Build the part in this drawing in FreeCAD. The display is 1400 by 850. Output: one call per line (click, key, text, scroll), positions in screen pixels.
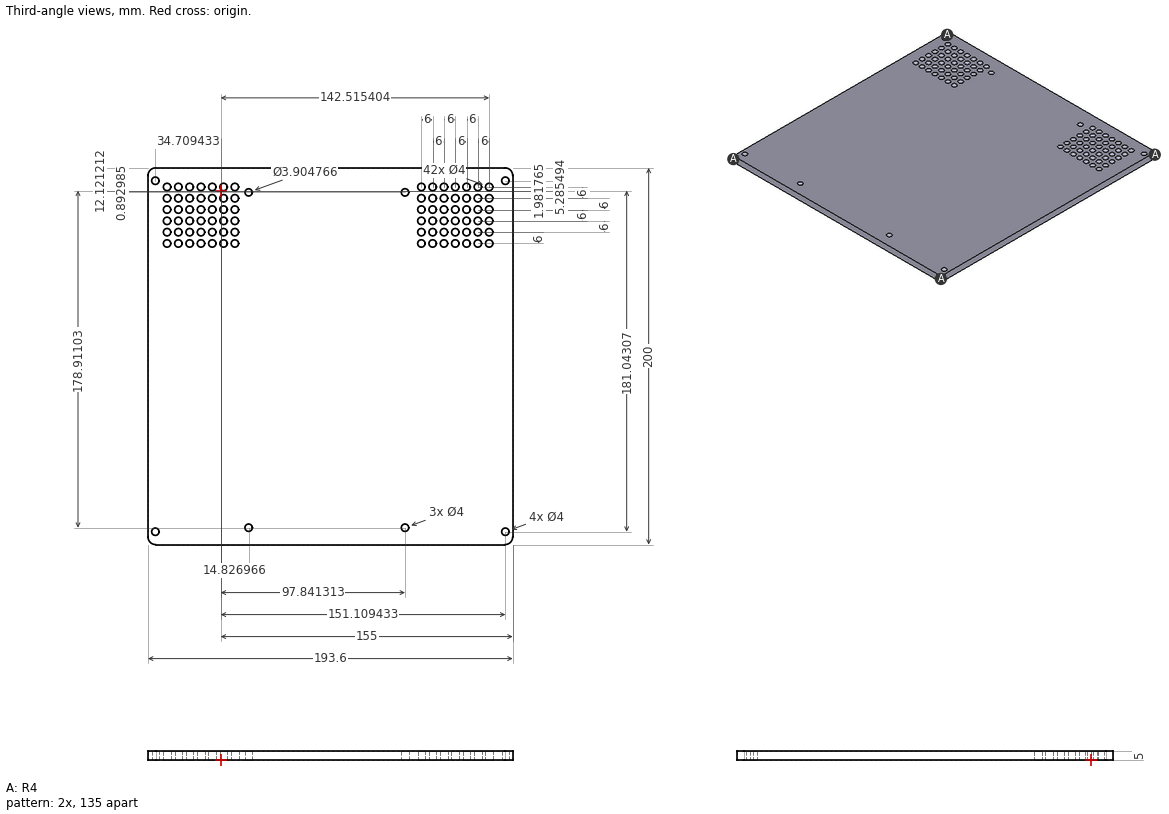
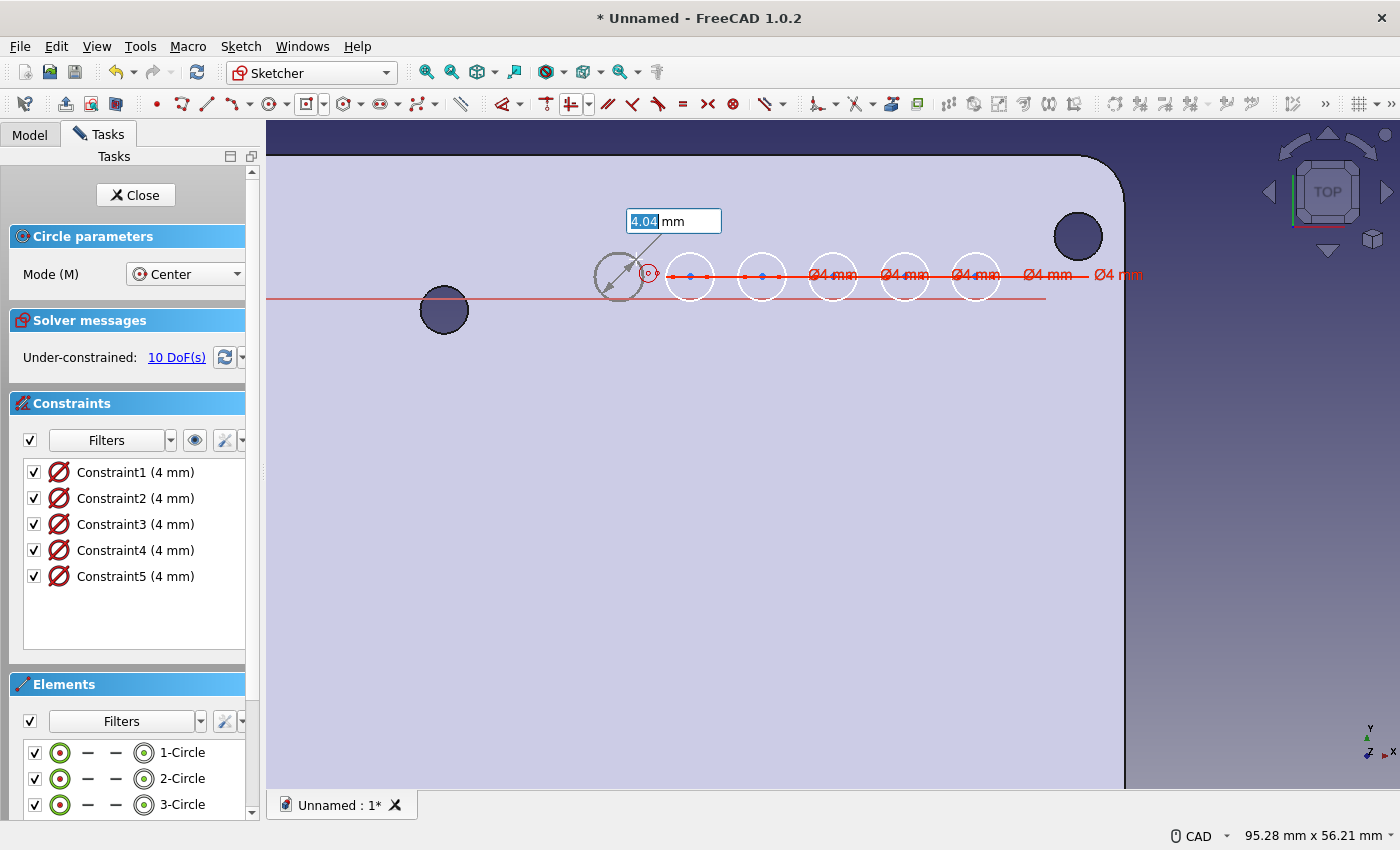
text(4)
key(Return)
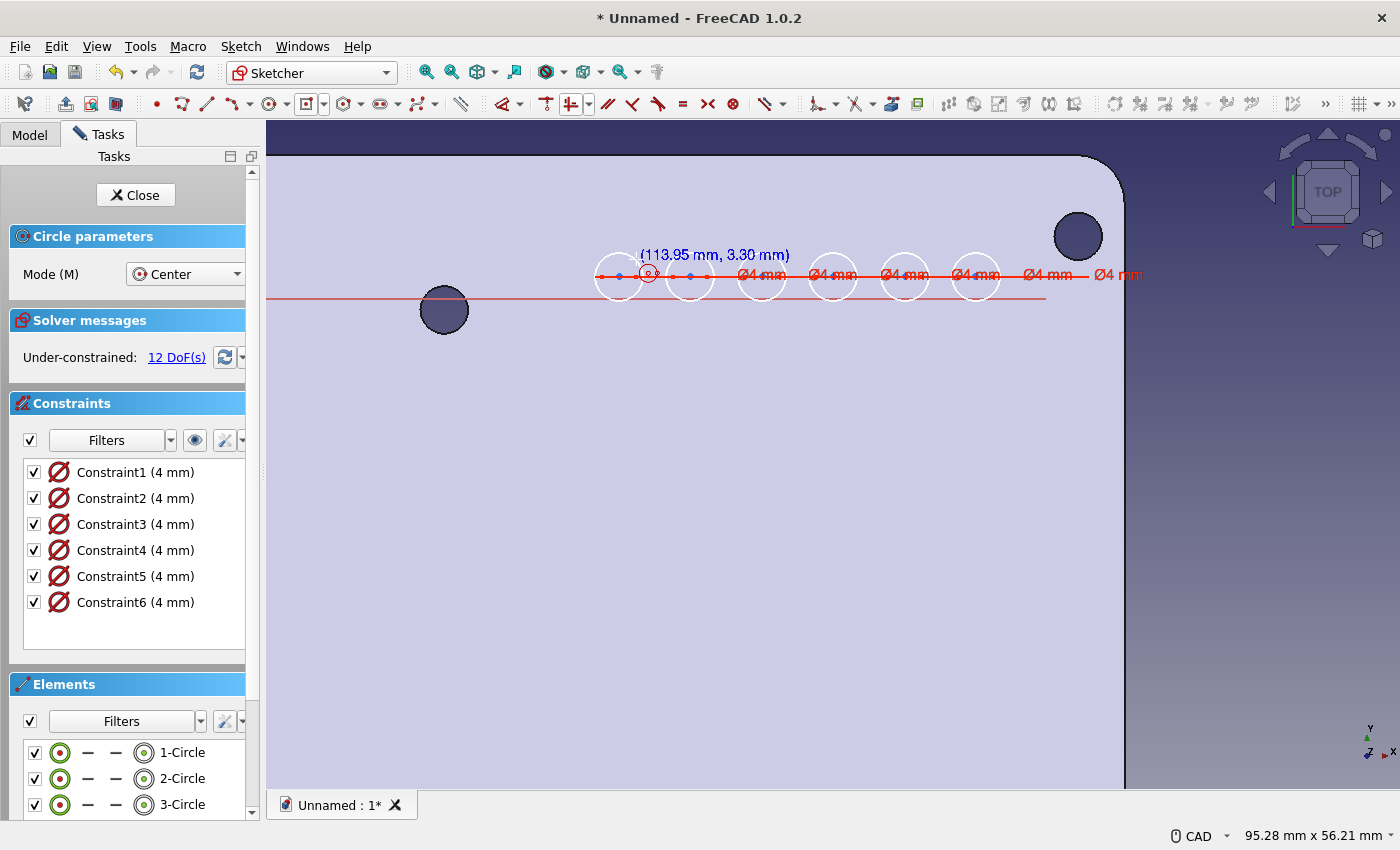
click(548, 276)
move(564, 259)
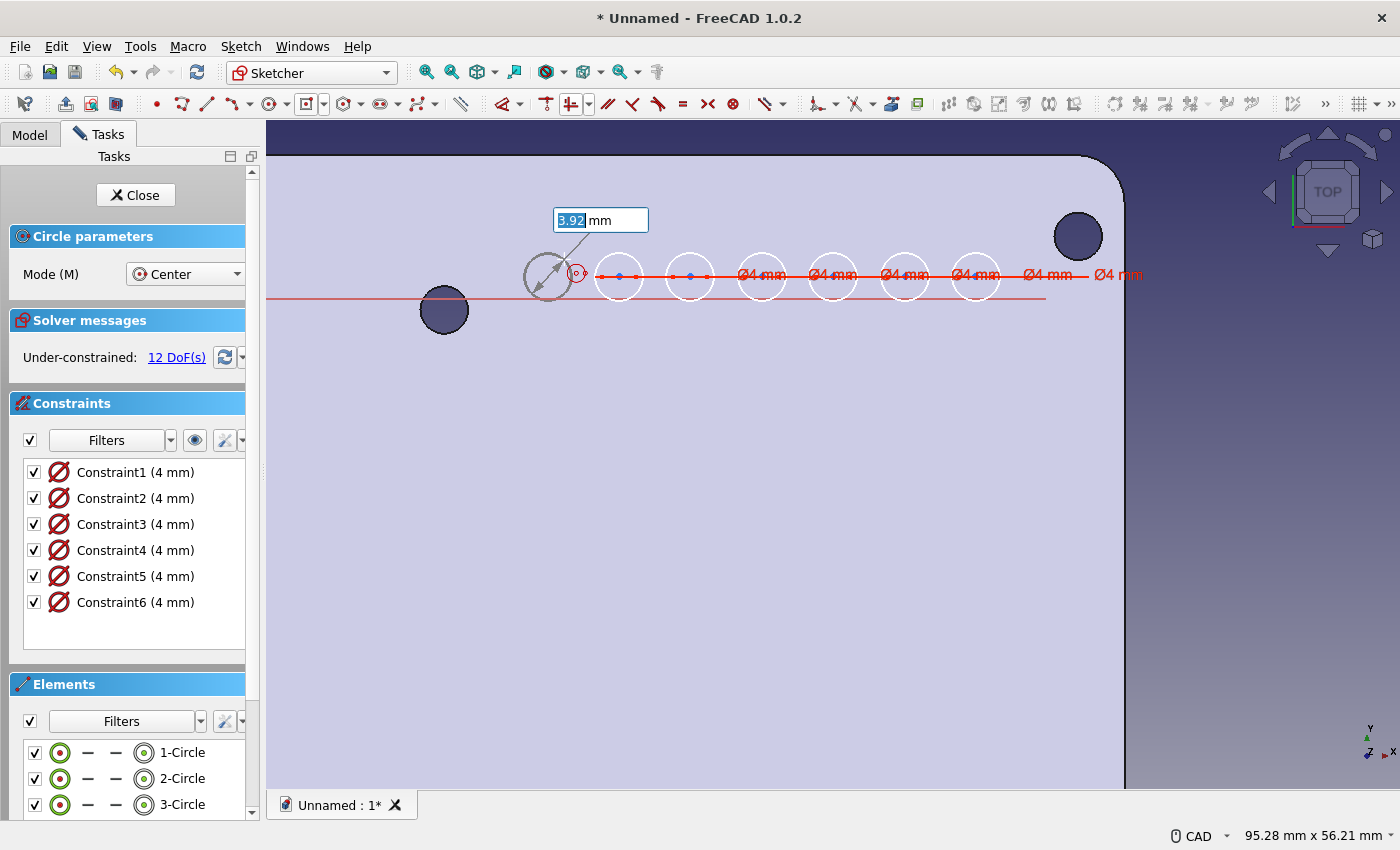
text(4)
key(Return)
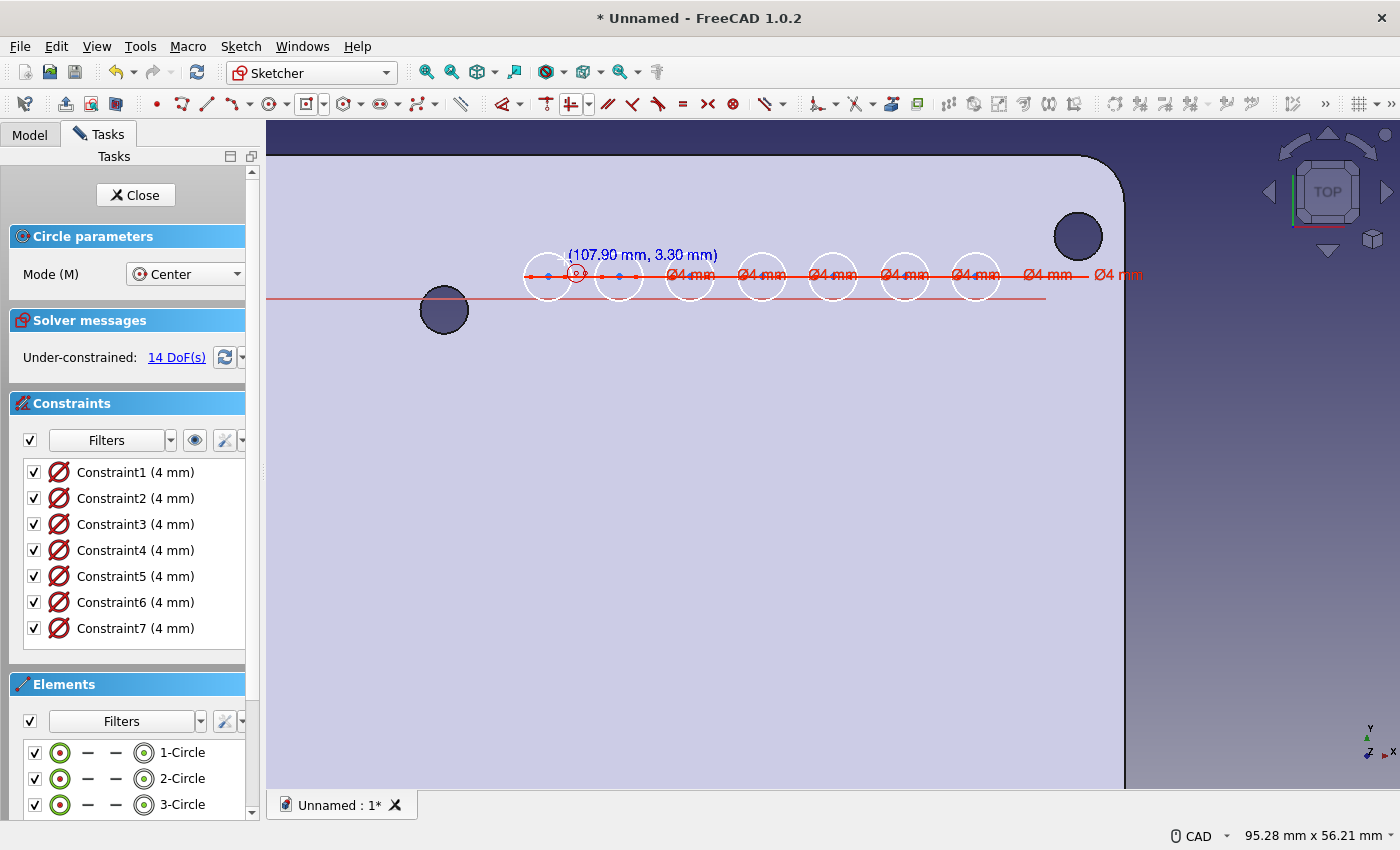
click(905, 347)
move(921, 330)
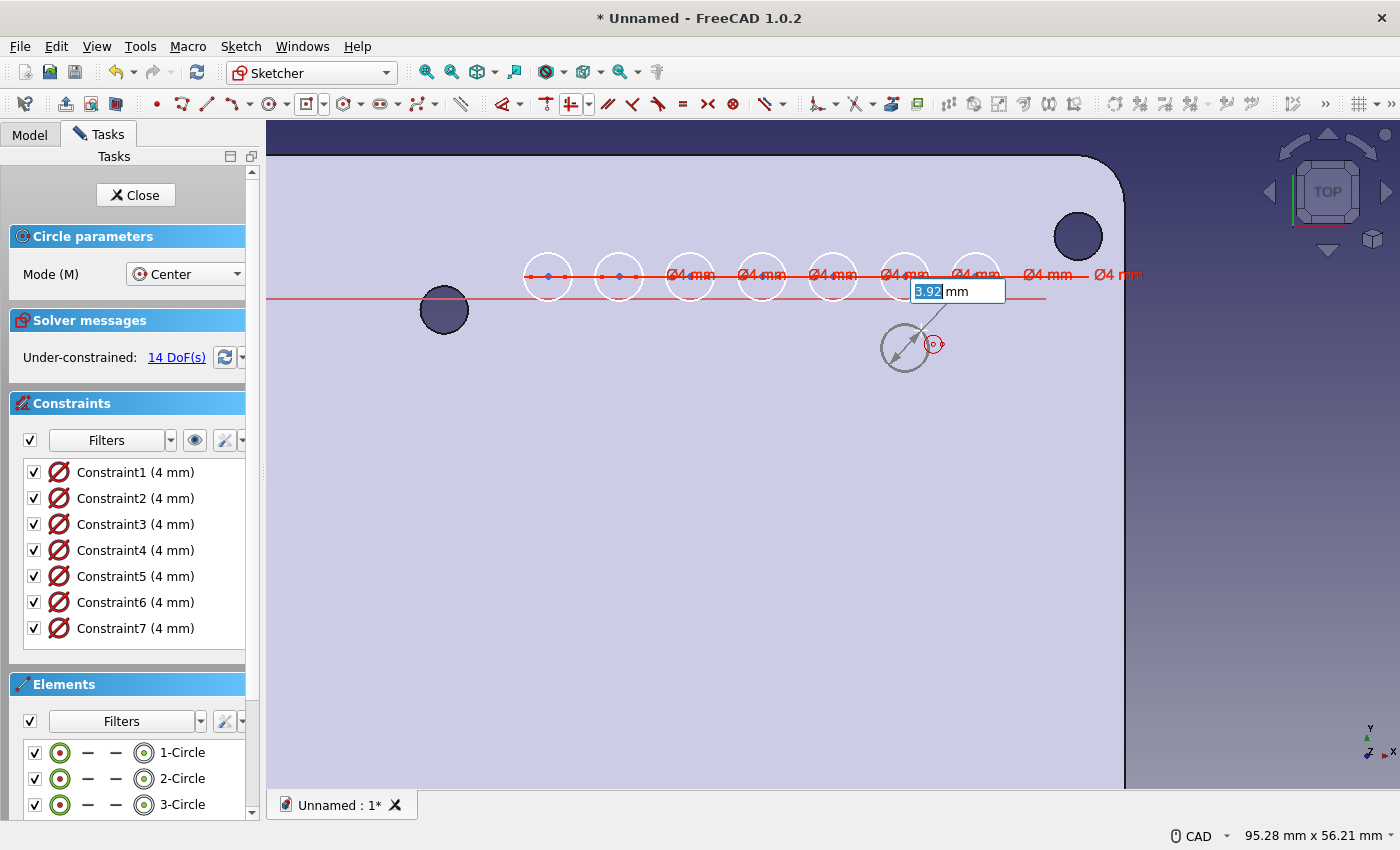
text(4)
key(Return)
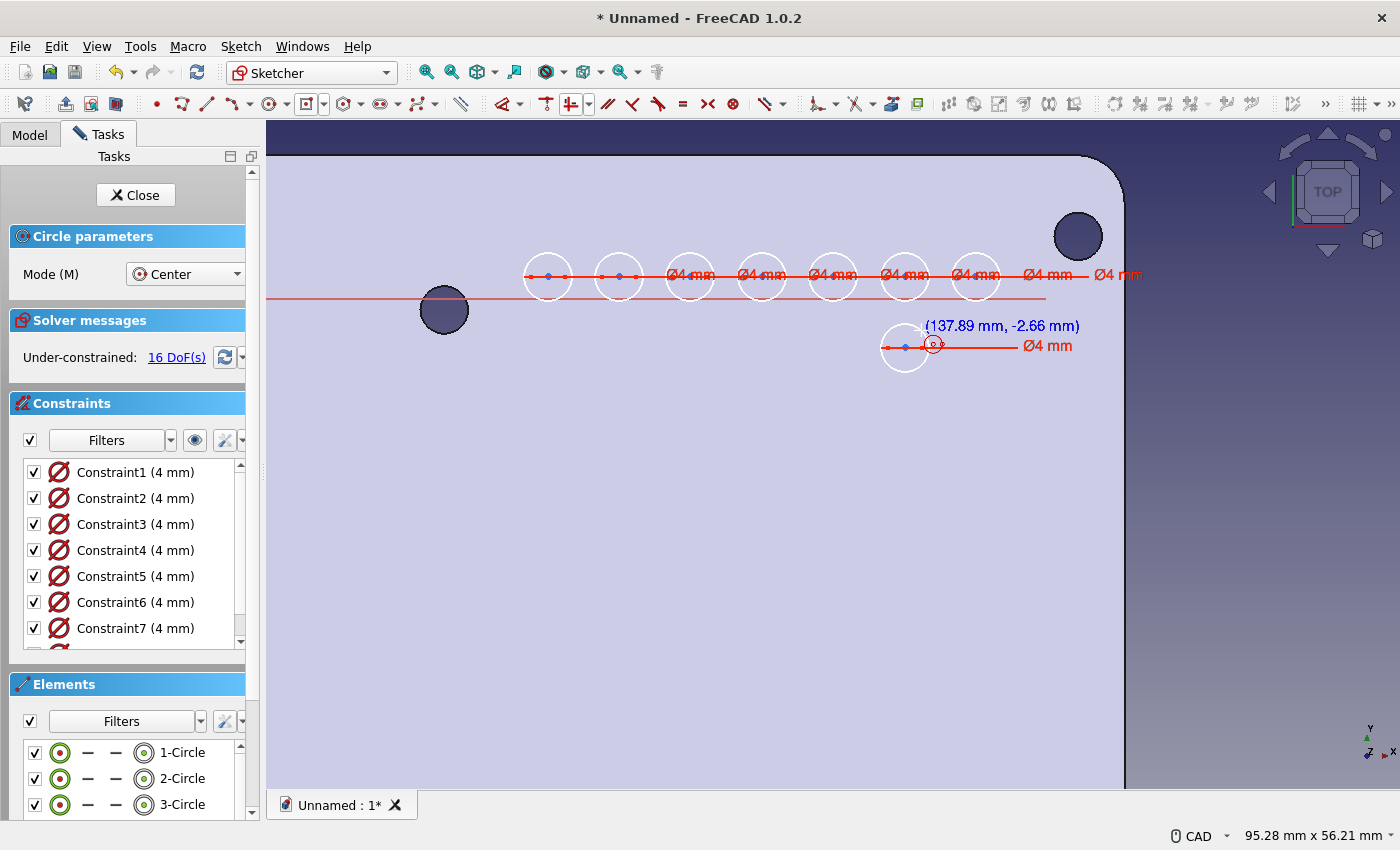
click(833, 347)
move(850, 330)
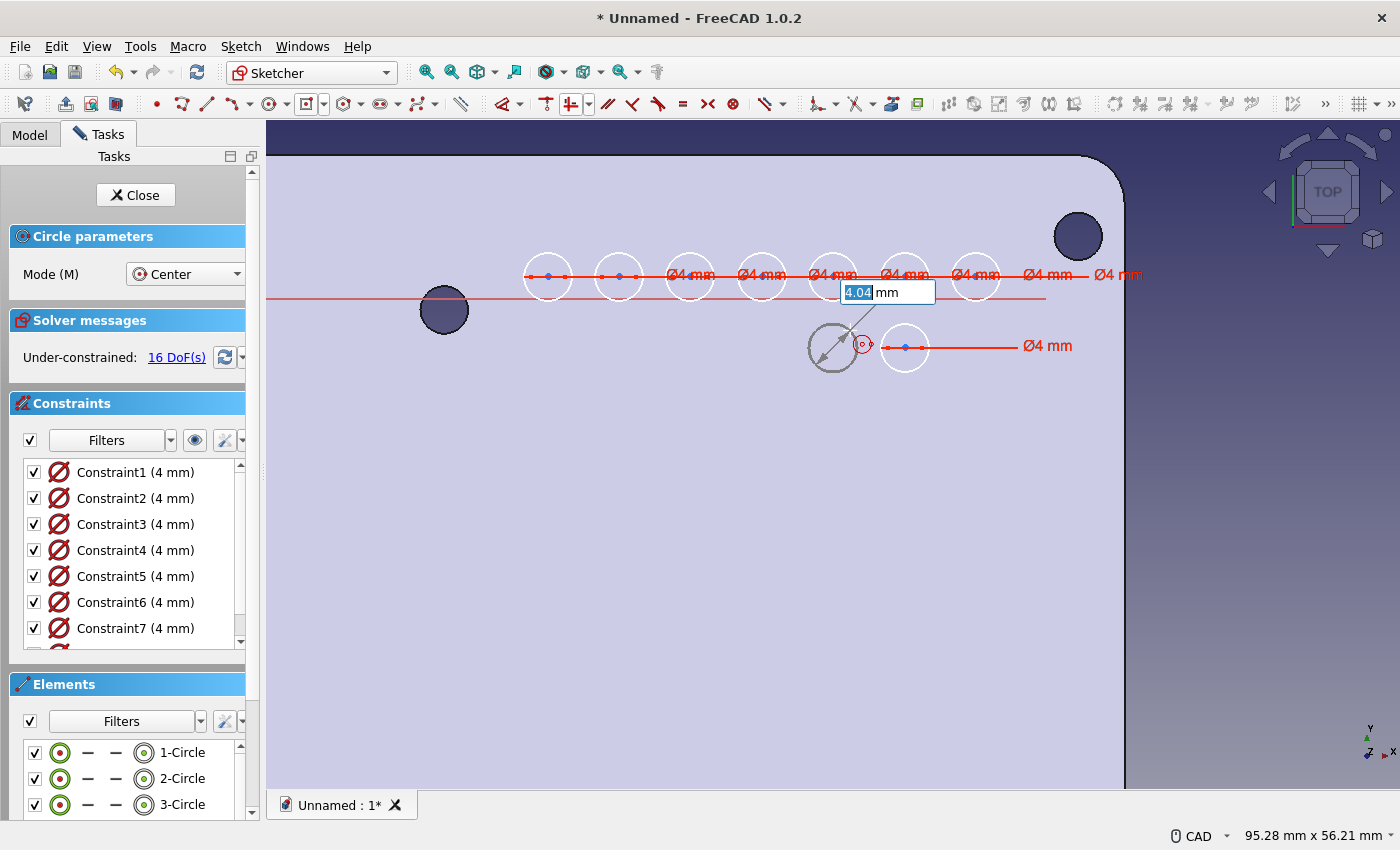
text(4)
key(Return)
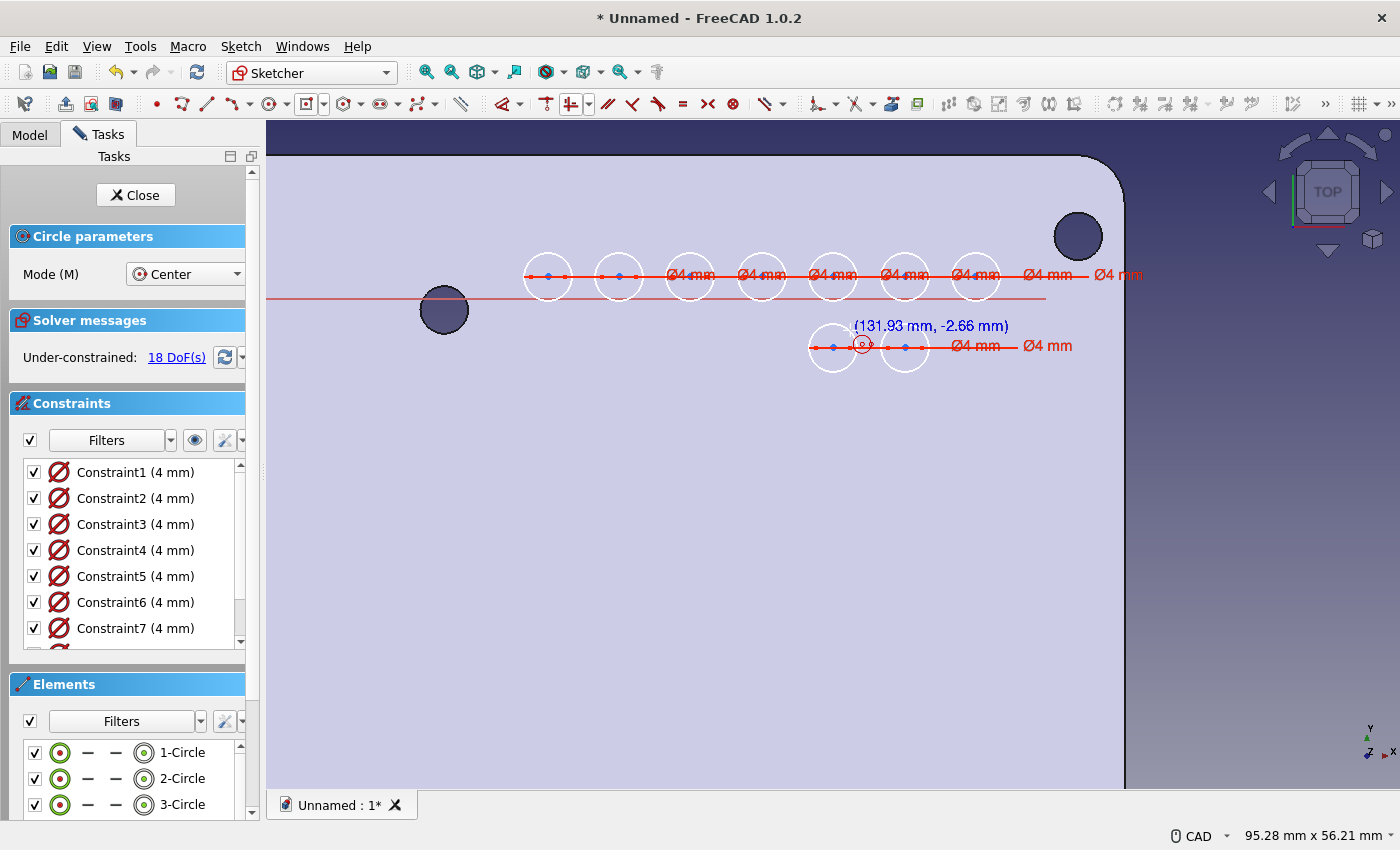
click(762, 347)
move(779, 330)